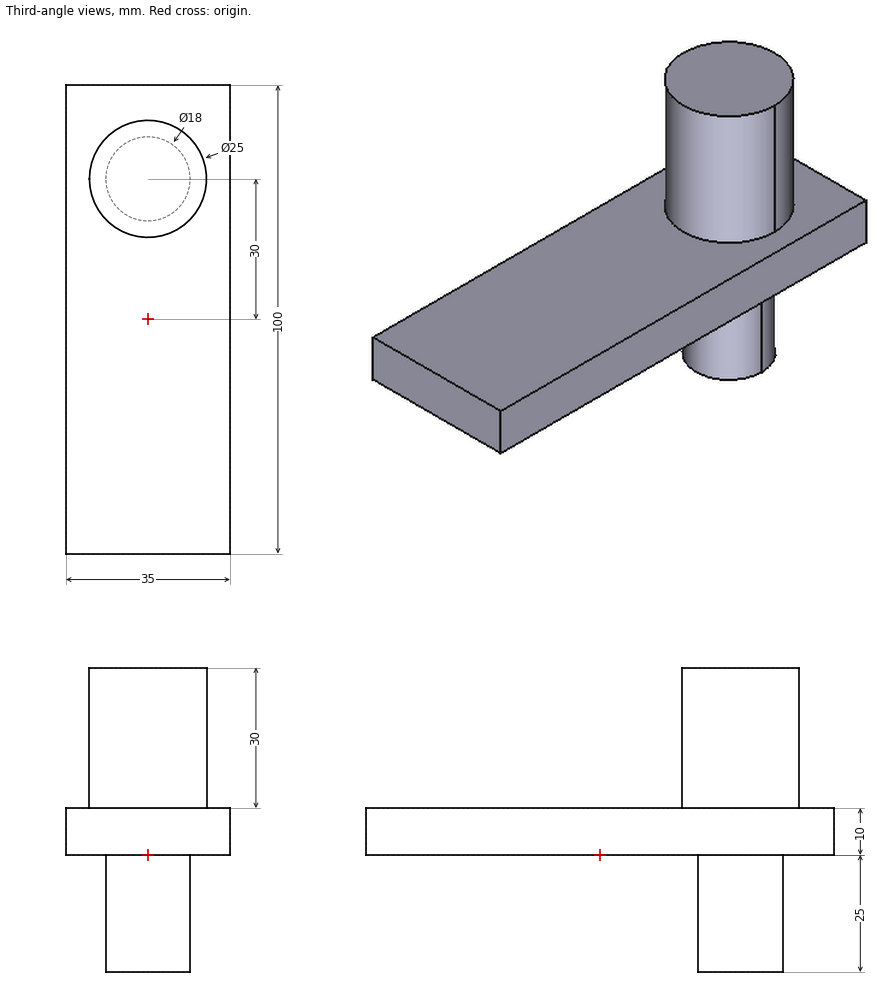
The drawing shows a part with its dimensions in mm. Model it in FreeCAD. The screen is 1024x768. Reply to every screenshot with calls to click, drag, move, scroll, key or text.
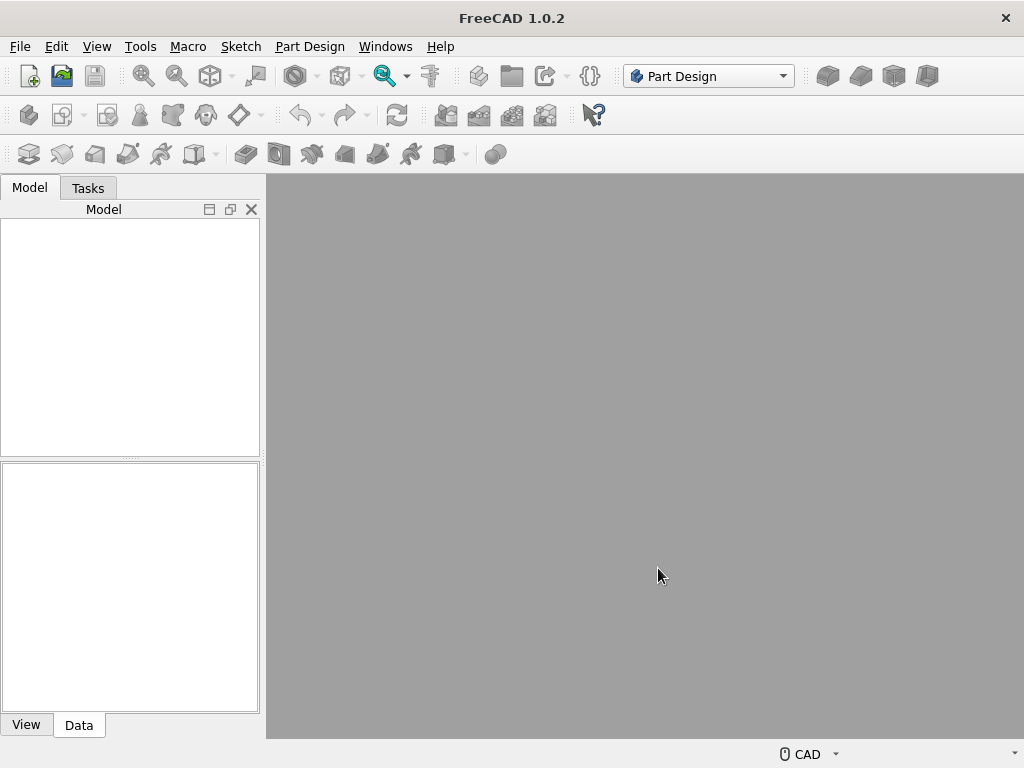
click(29, 76)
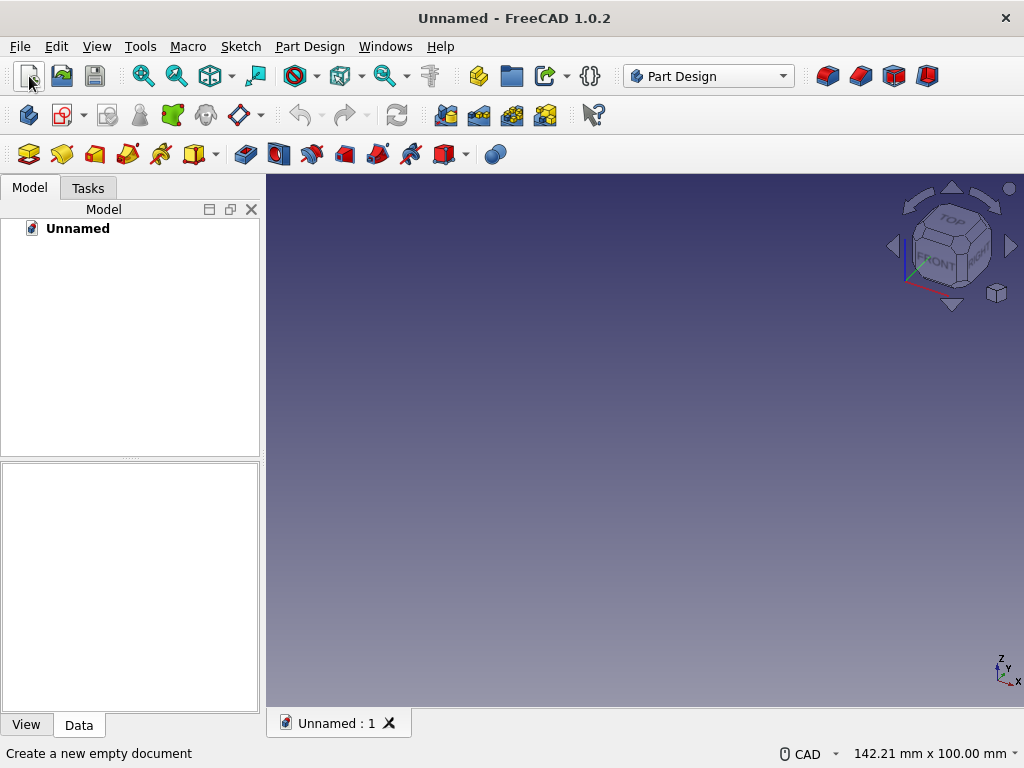
click(62, 116)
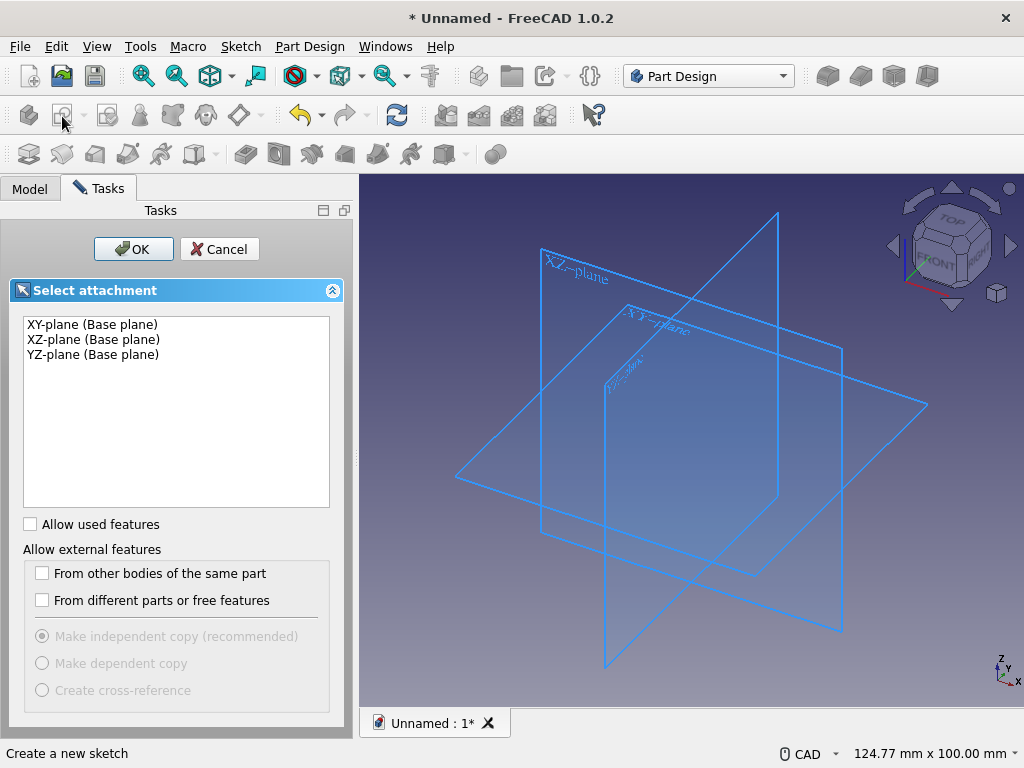
click(84, 324)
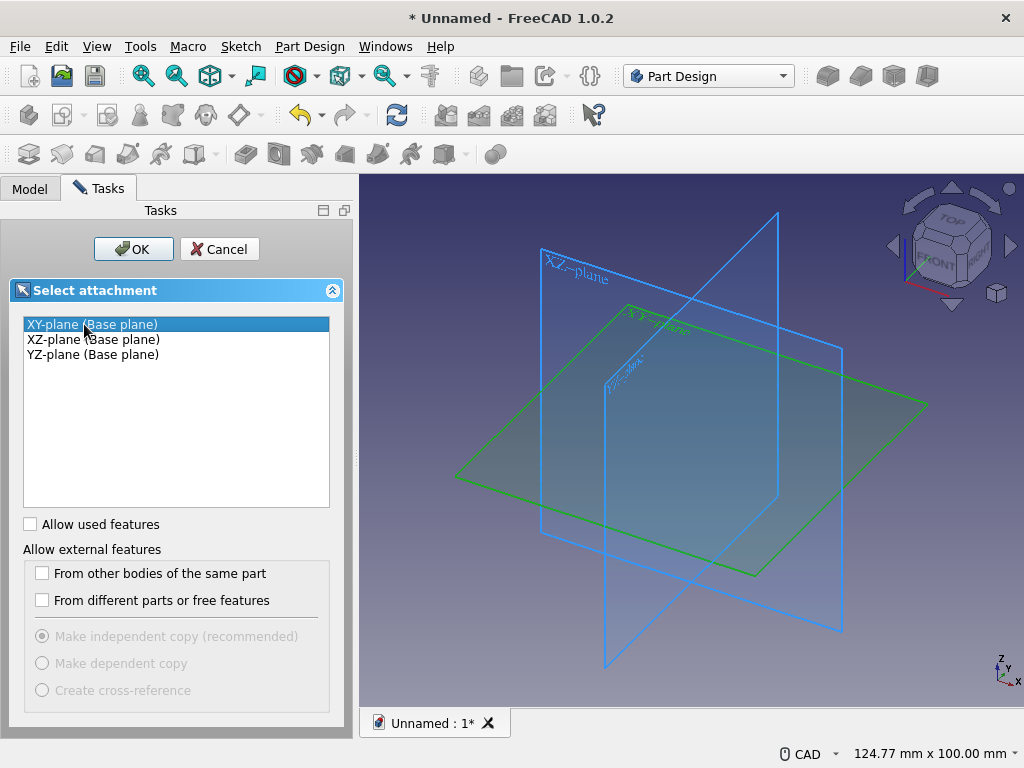
click(134, 249)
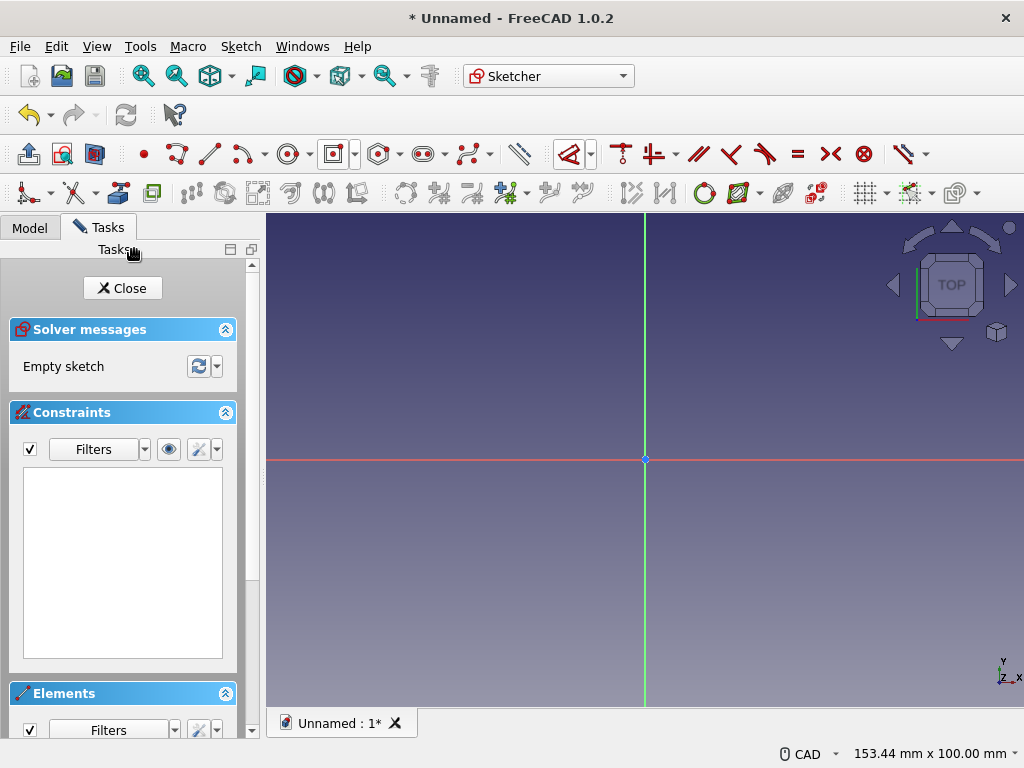
scroll(437, 460, down, 2)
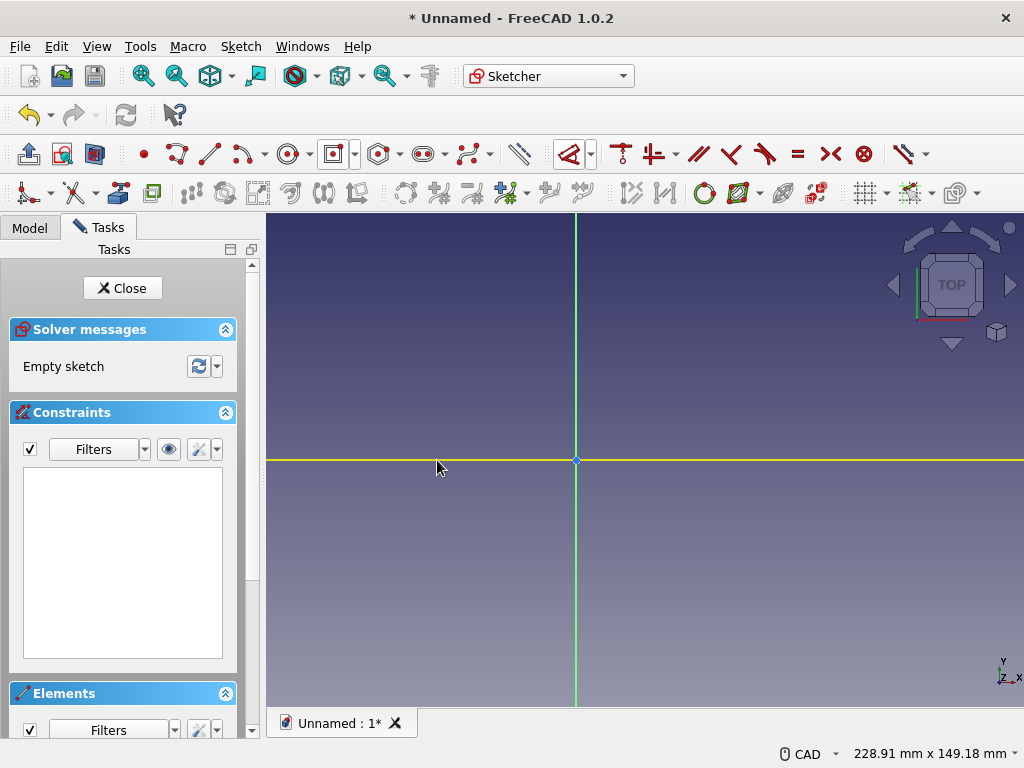
click(332, 154)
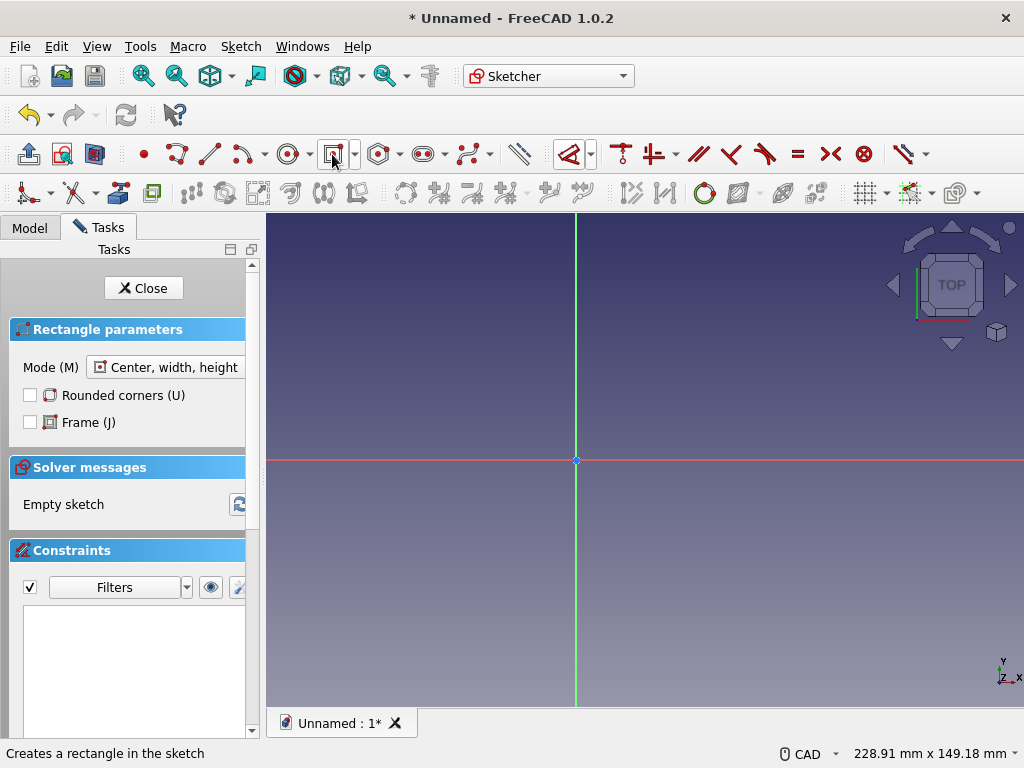
click(577, 460)
click(634, 295)
key(Escape)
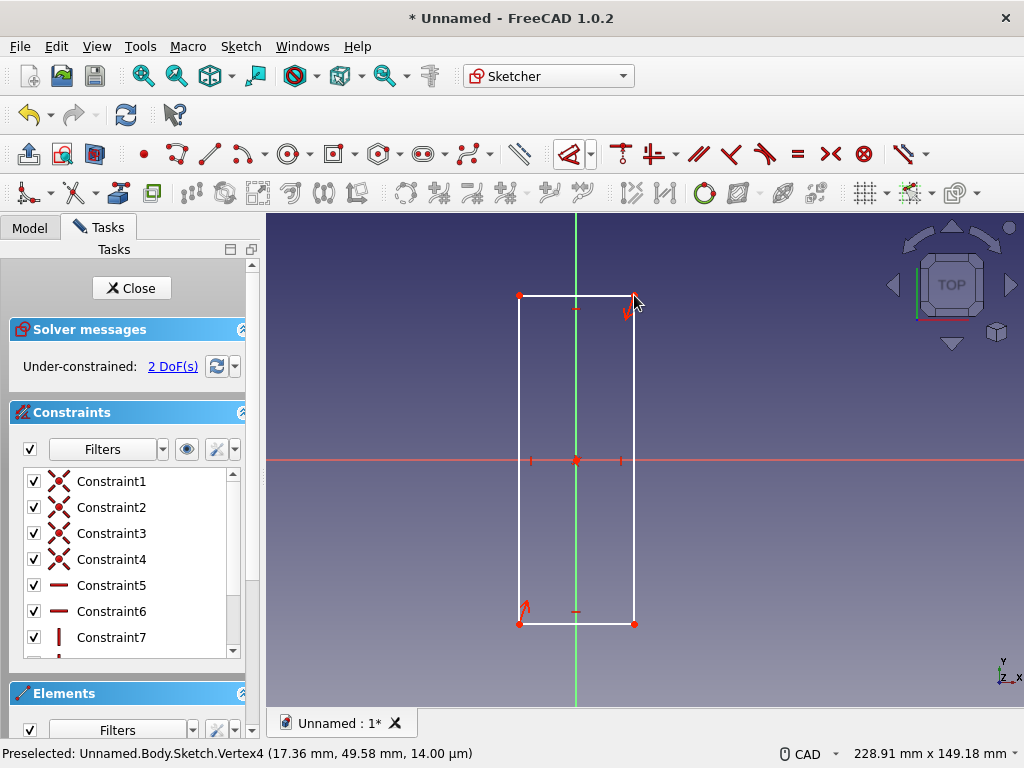
click(568, 154)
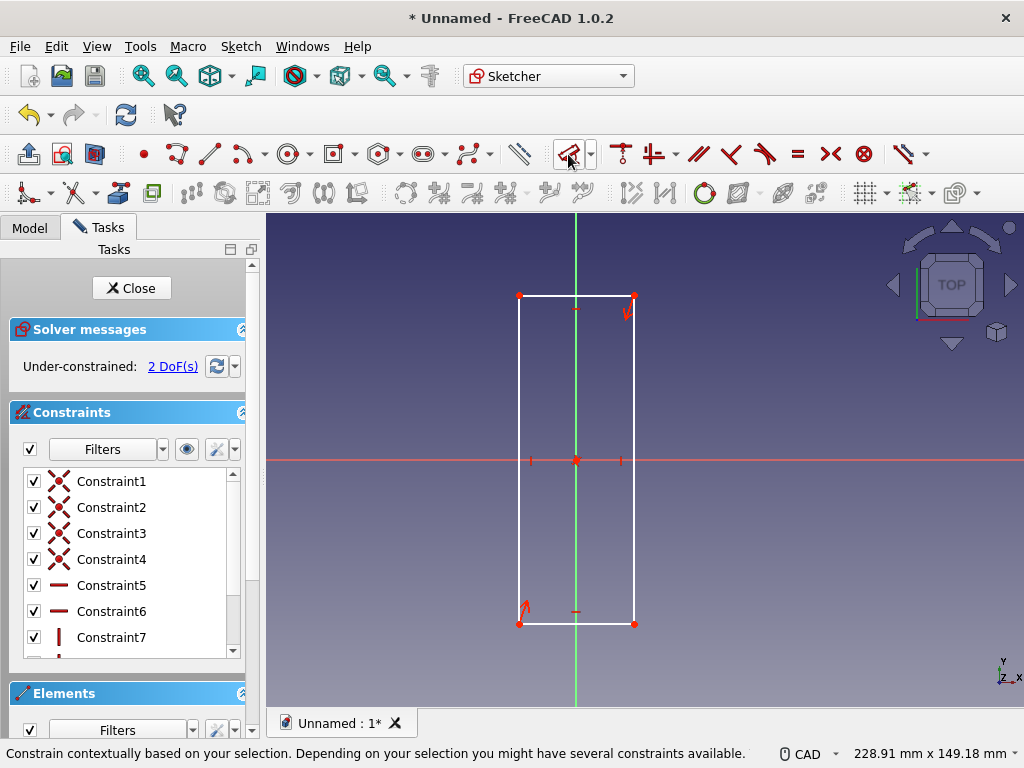
click(554, 624)
click(550, 658)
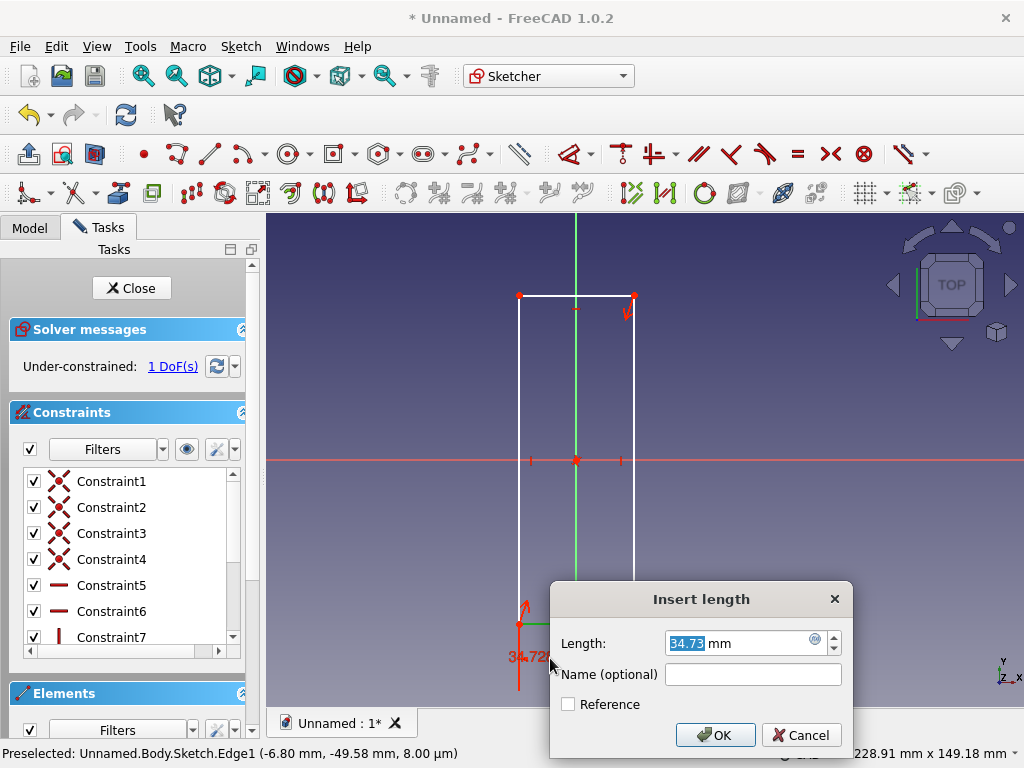
text(35)
key(Return)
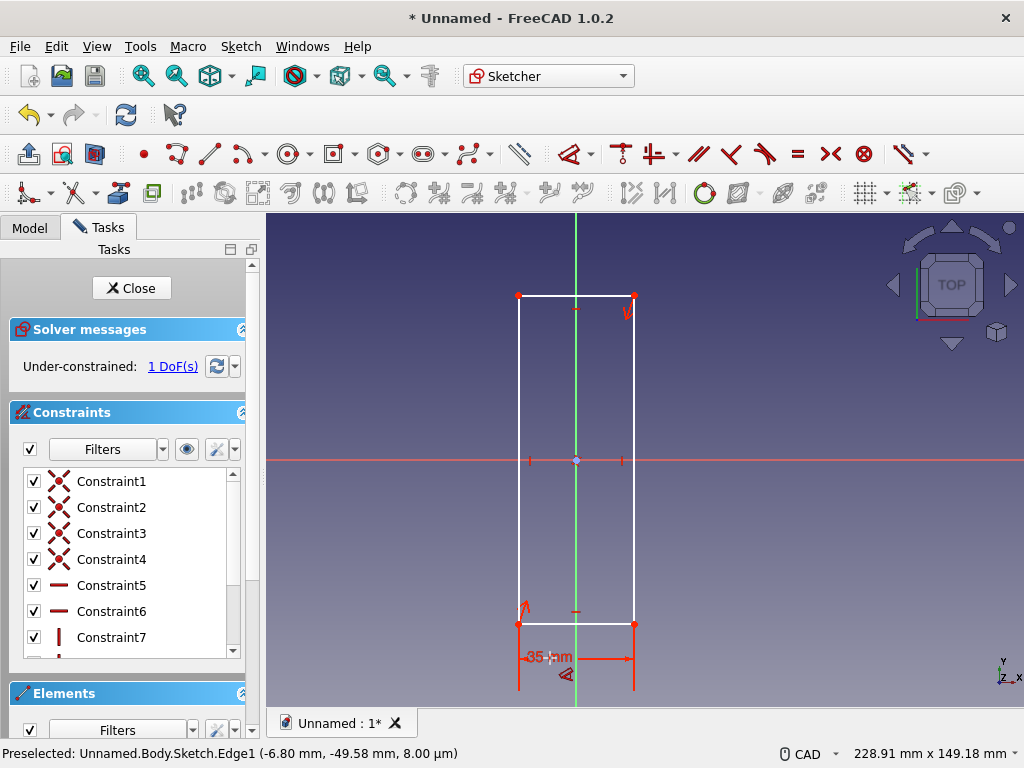
click(634, 526)
click(668, 385)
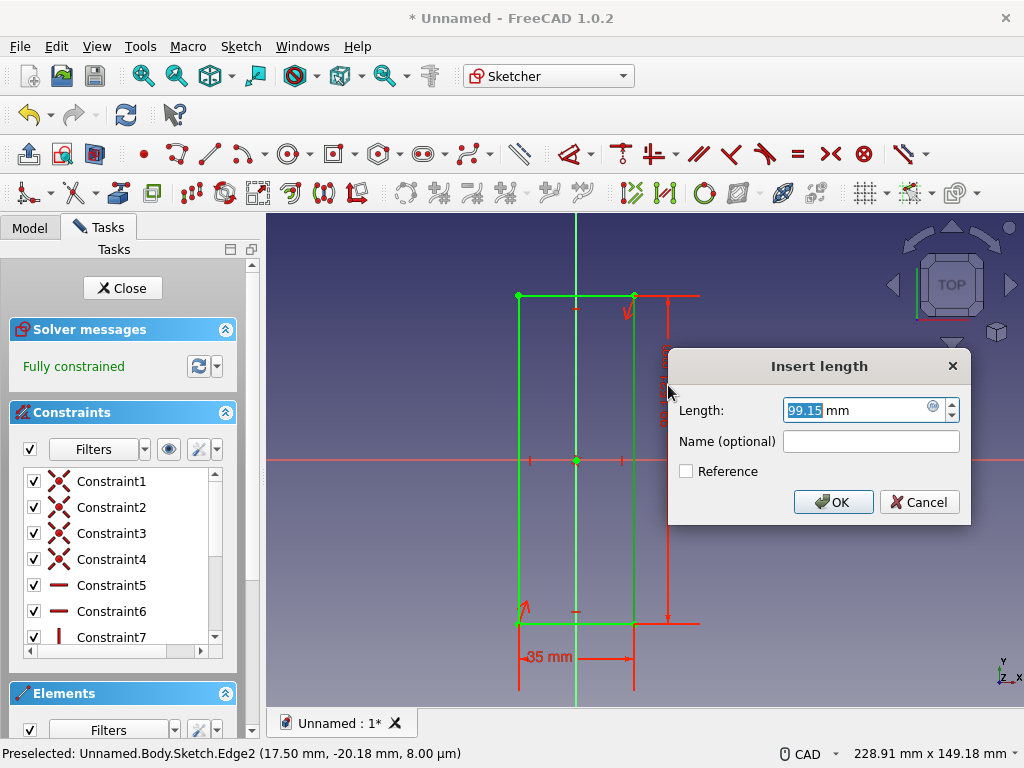
text(100)
key(Return)
key(Escape)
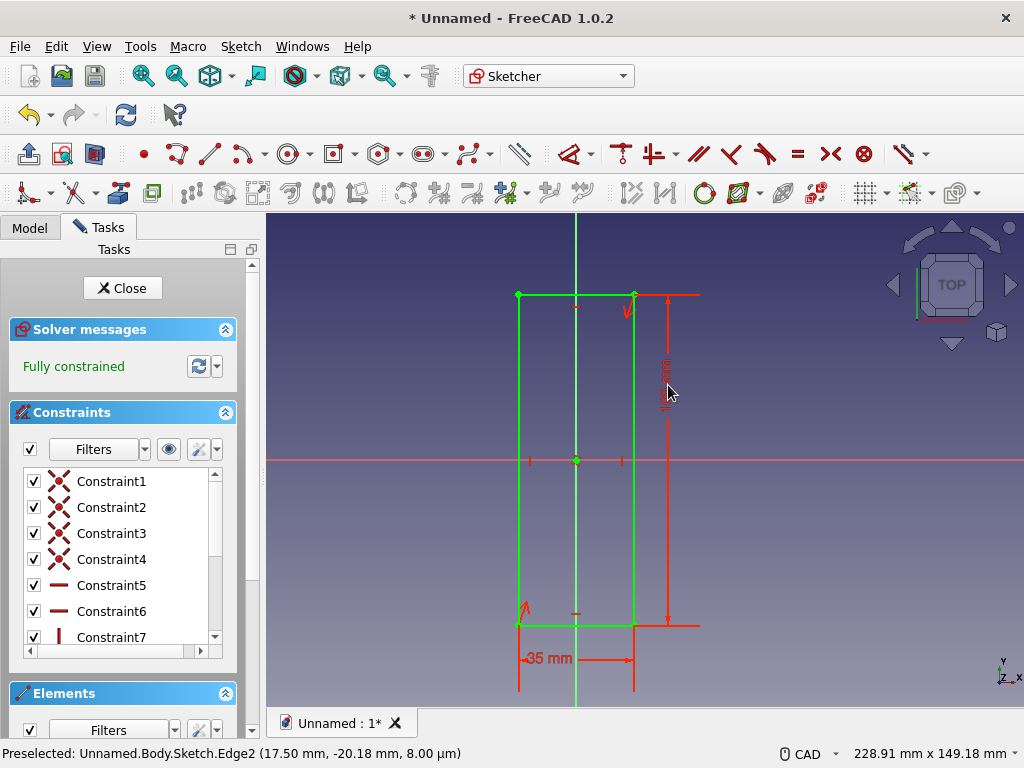
click(123, 288)